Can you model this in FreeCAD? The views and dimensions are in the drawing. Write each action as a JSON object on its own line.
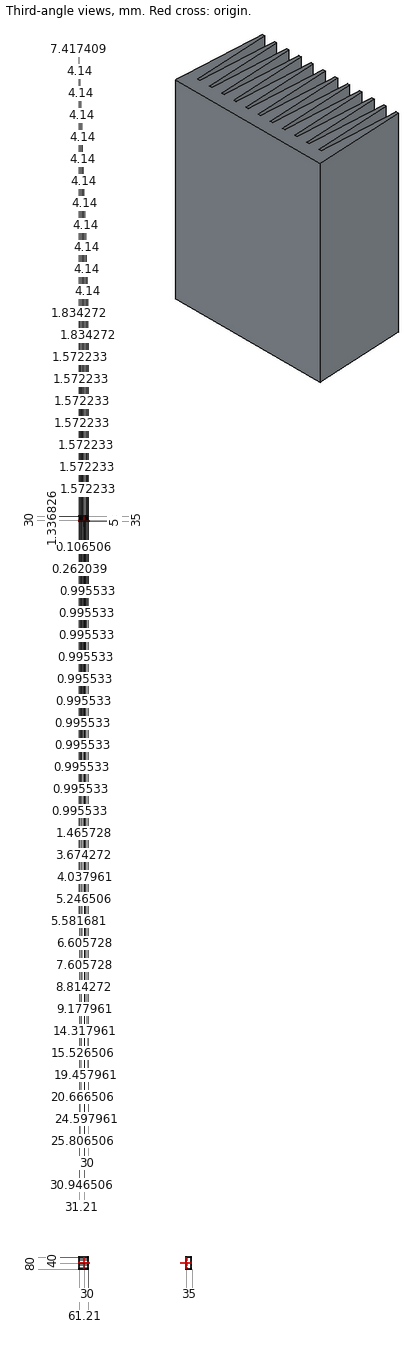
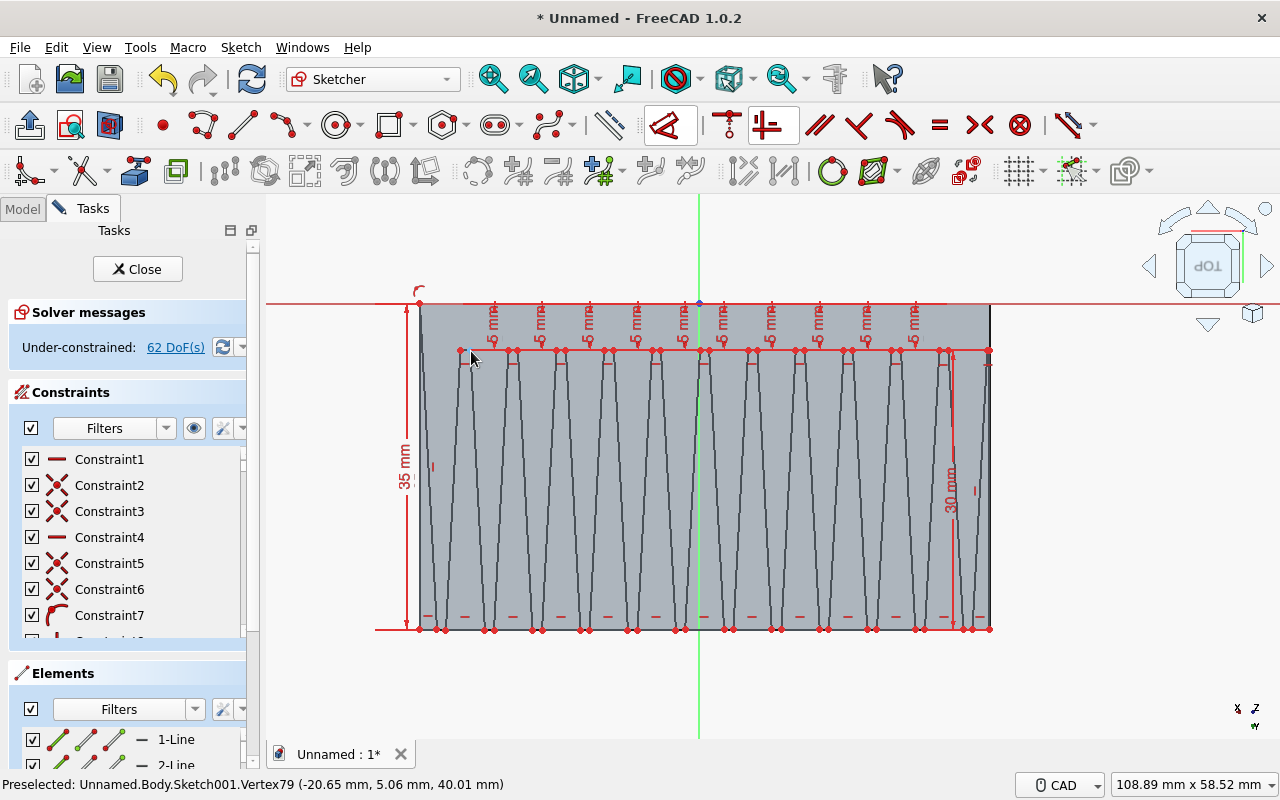
{"action": "scroll", "coordinate": [939, 351], "scroll_direction": "up", "scroll_amount": 2}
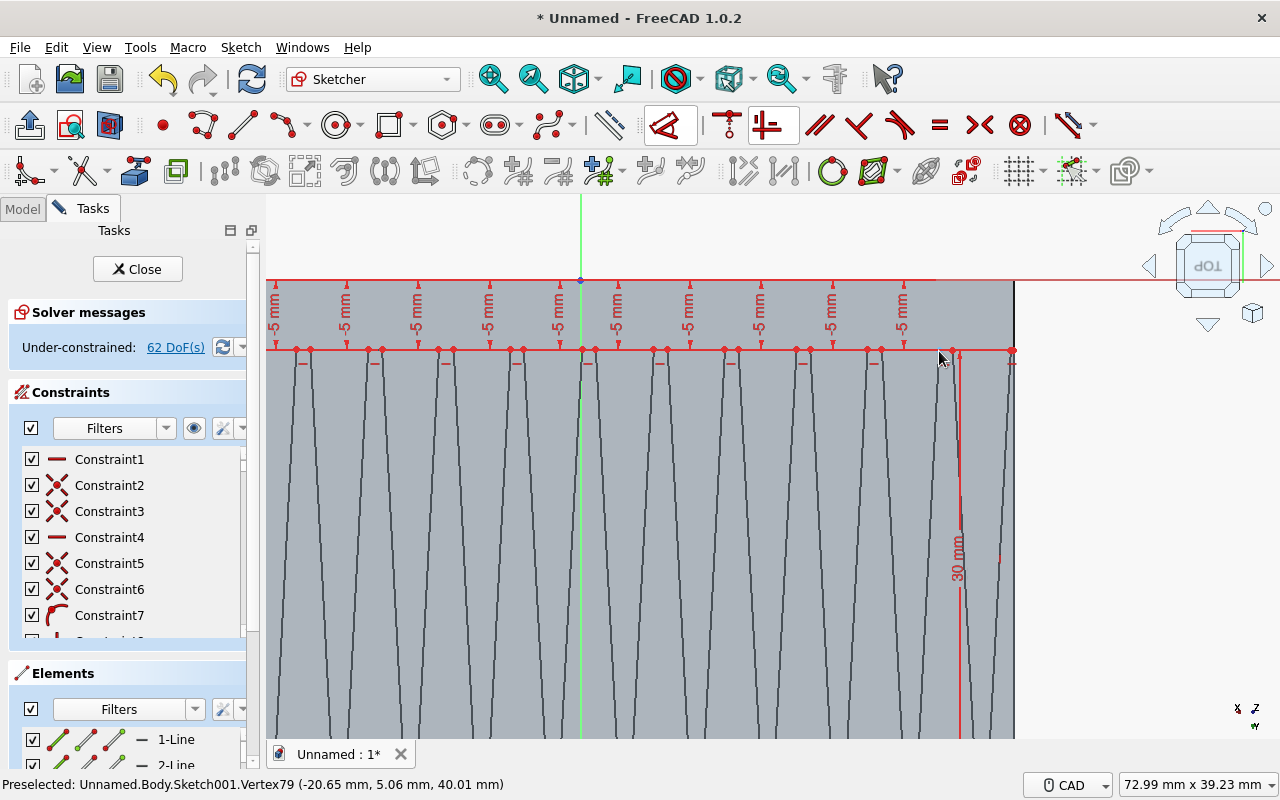
{"action": "left_click", "coordinate": [939, 350]}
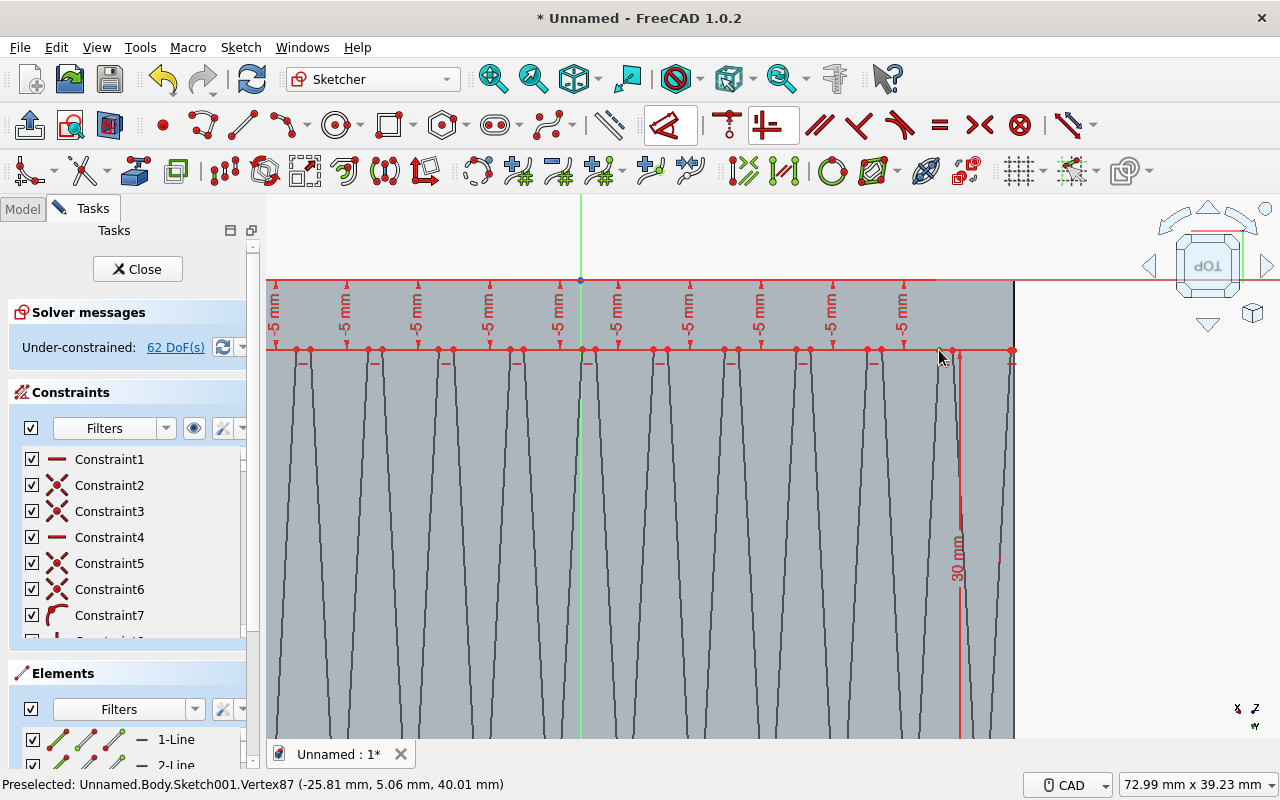
{"action": "key", "text": "i"}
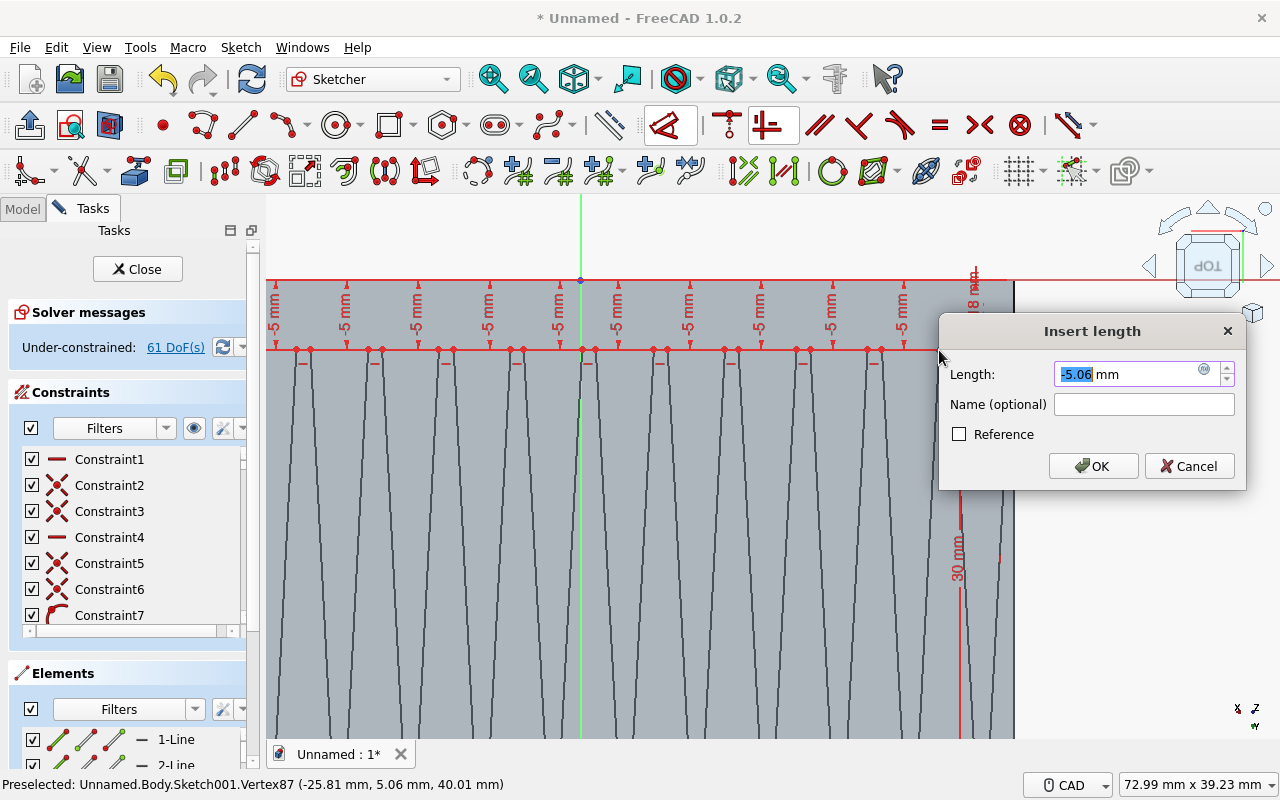
{"action": "type", "text": "-5"}
{"action": "key", "text": "Return"}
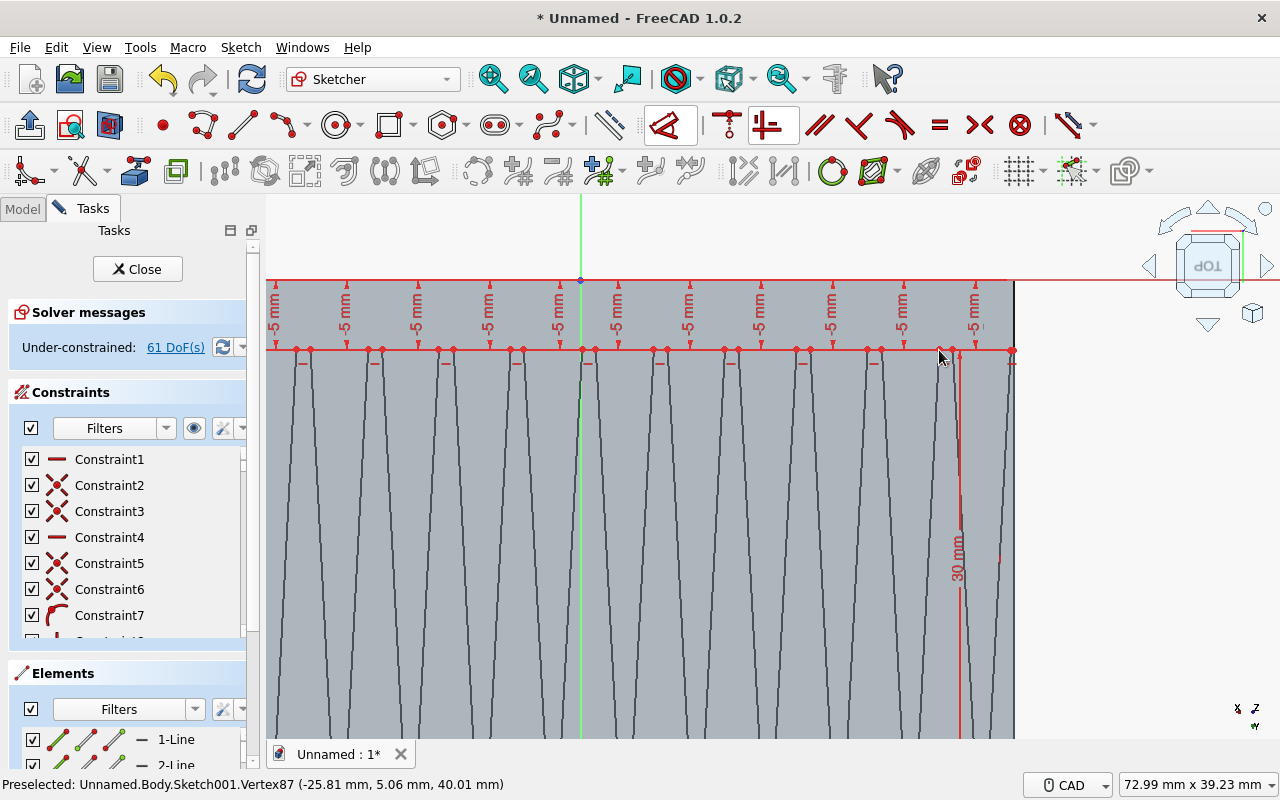
{"action": "scroll", "coordinate": [1011, 350], "scroll_direction": "up", "scroll_amount": 7}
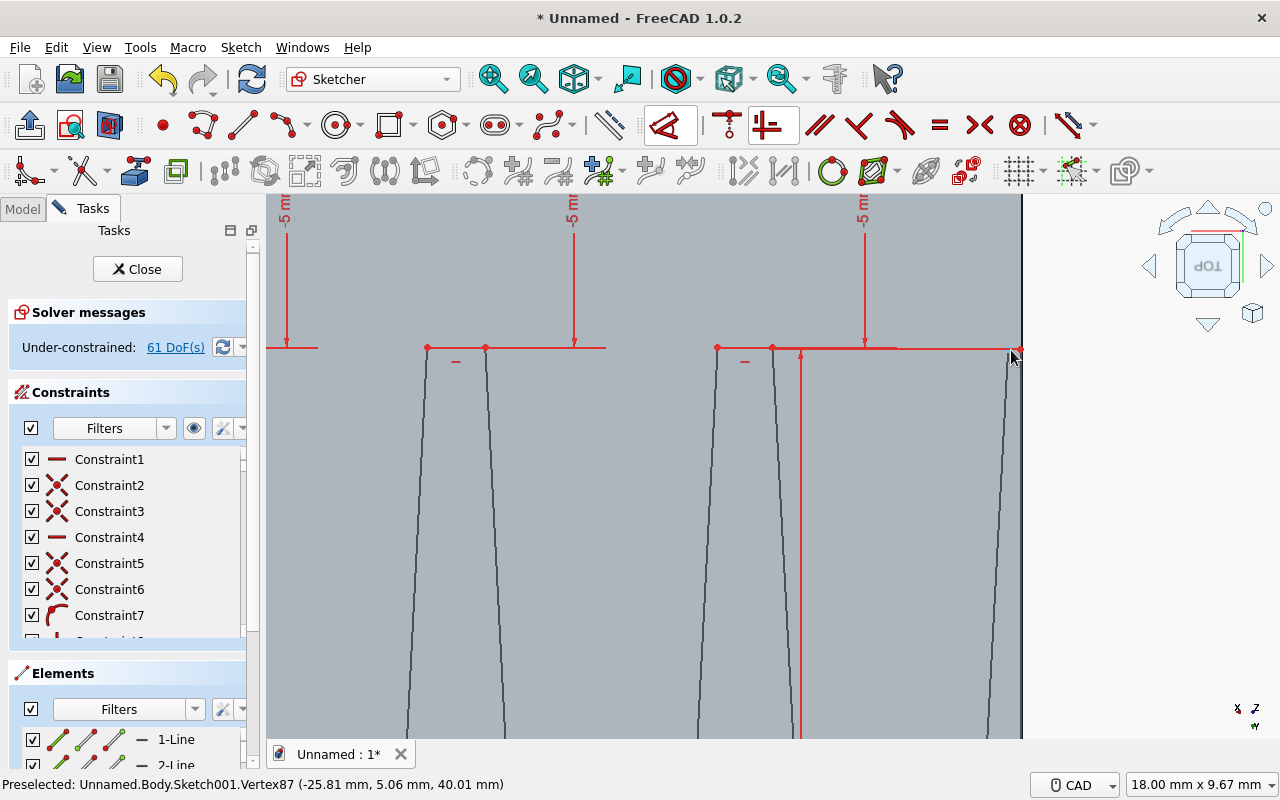
{"action": "left_click", "coordinate": [1008, 349]}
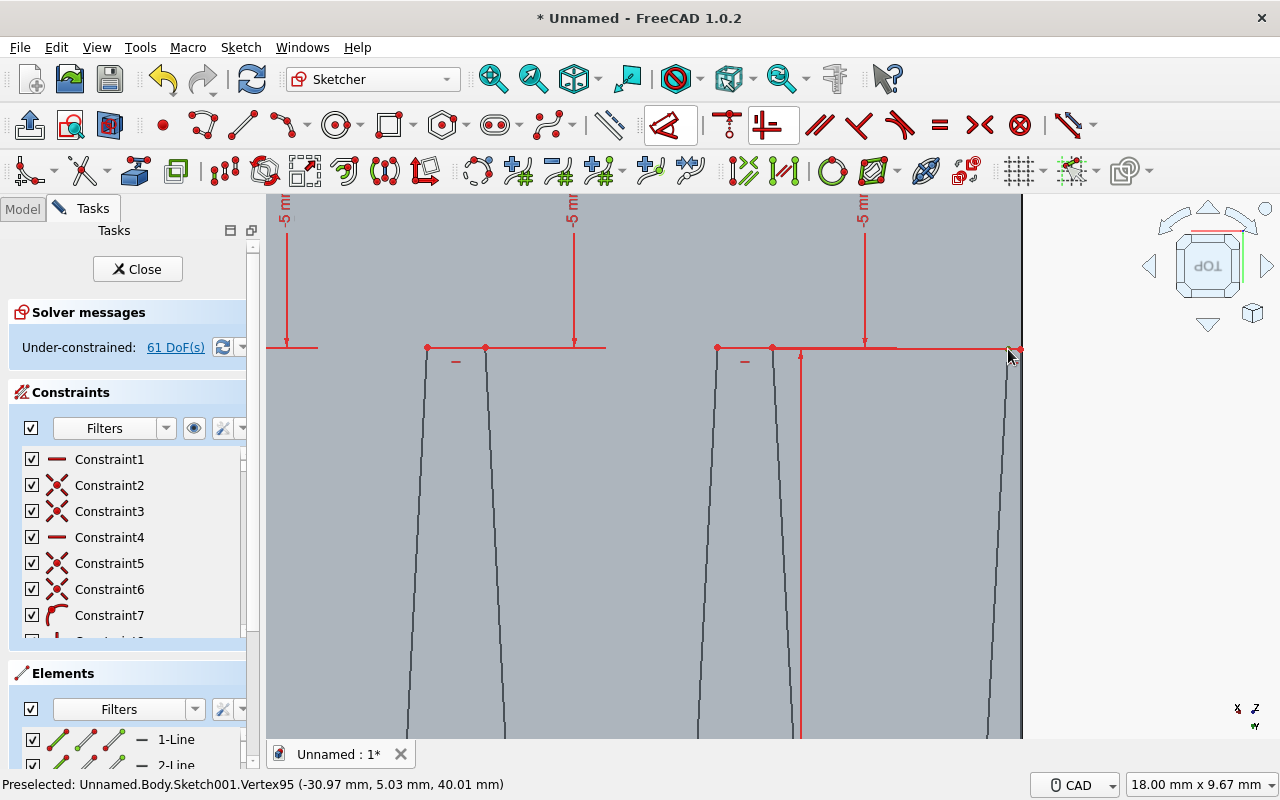
{"action": "key", "text": "i"}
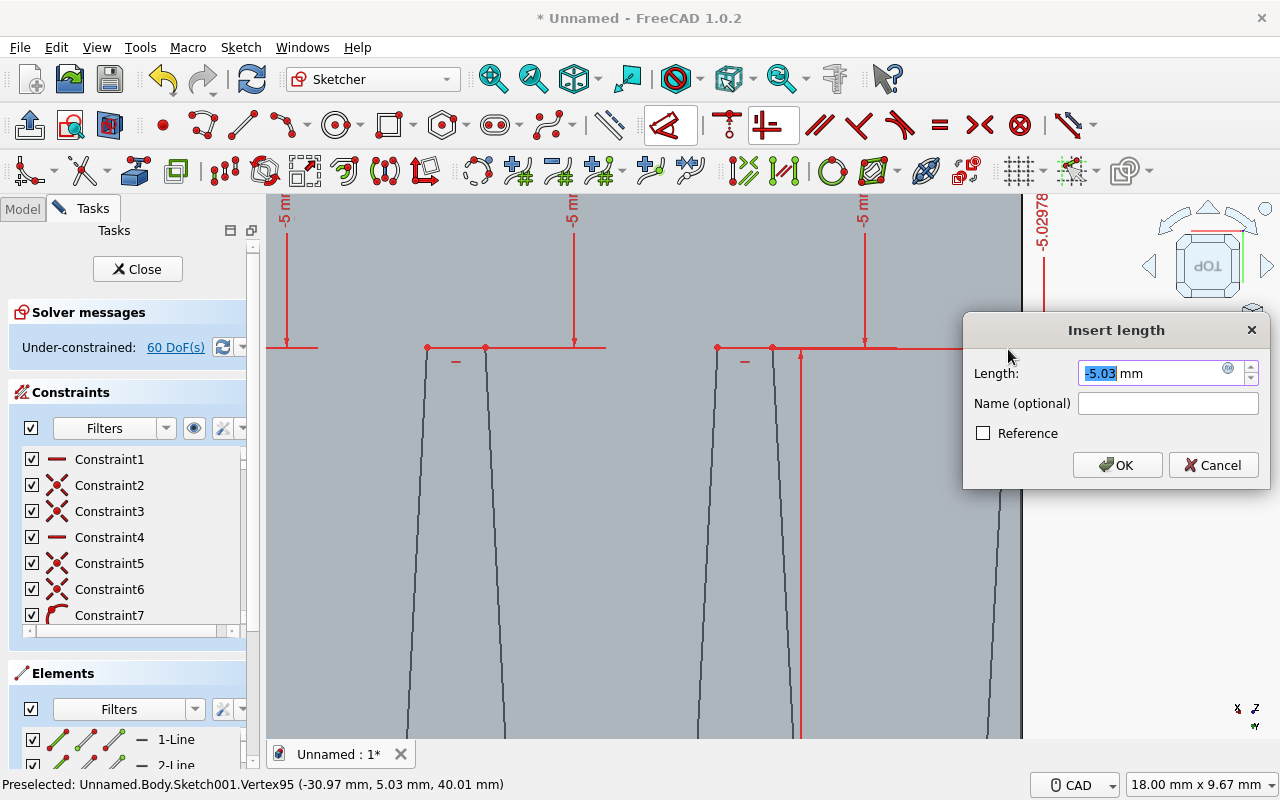
{"action": "type", "text": "-5"}
{"action": "key", "text": "Return"}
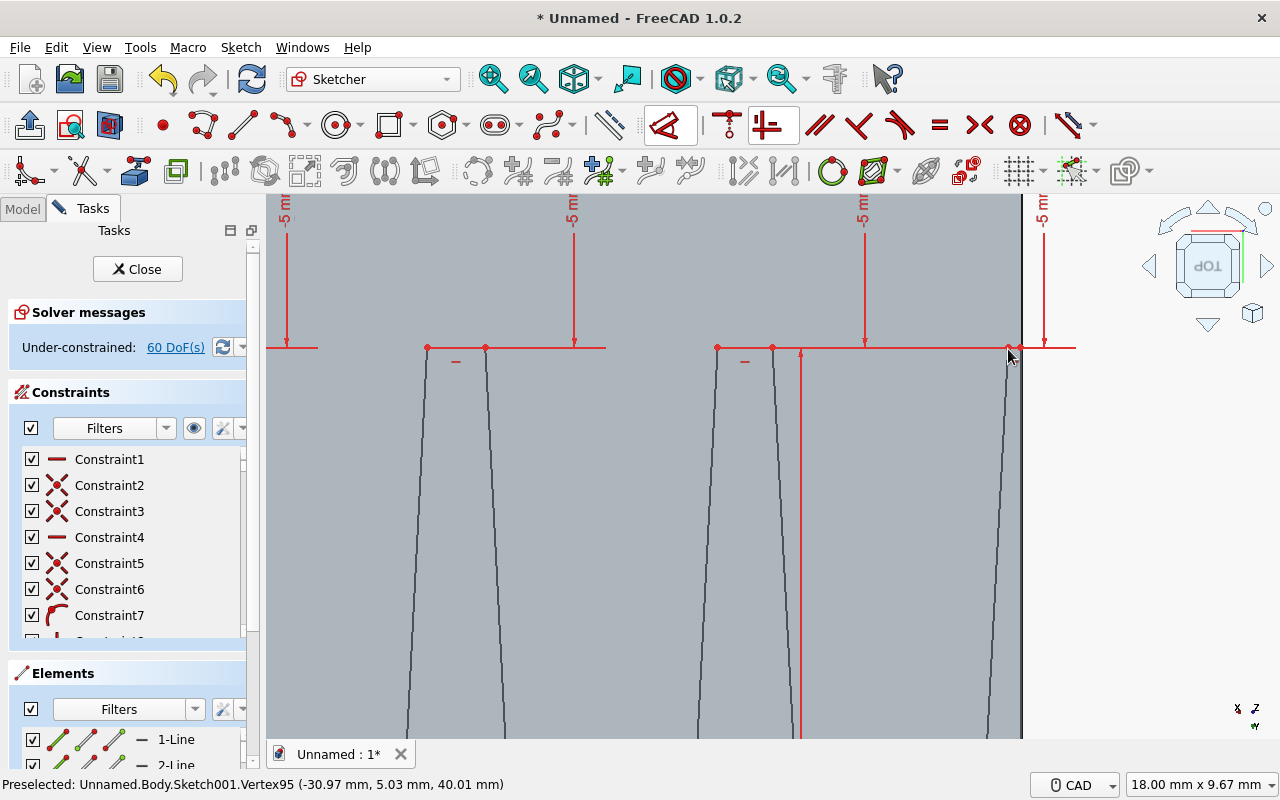
{"action": "scroll", "coordinate": [983, 351], "scroll_direction": "down", "scroll_amount": 9}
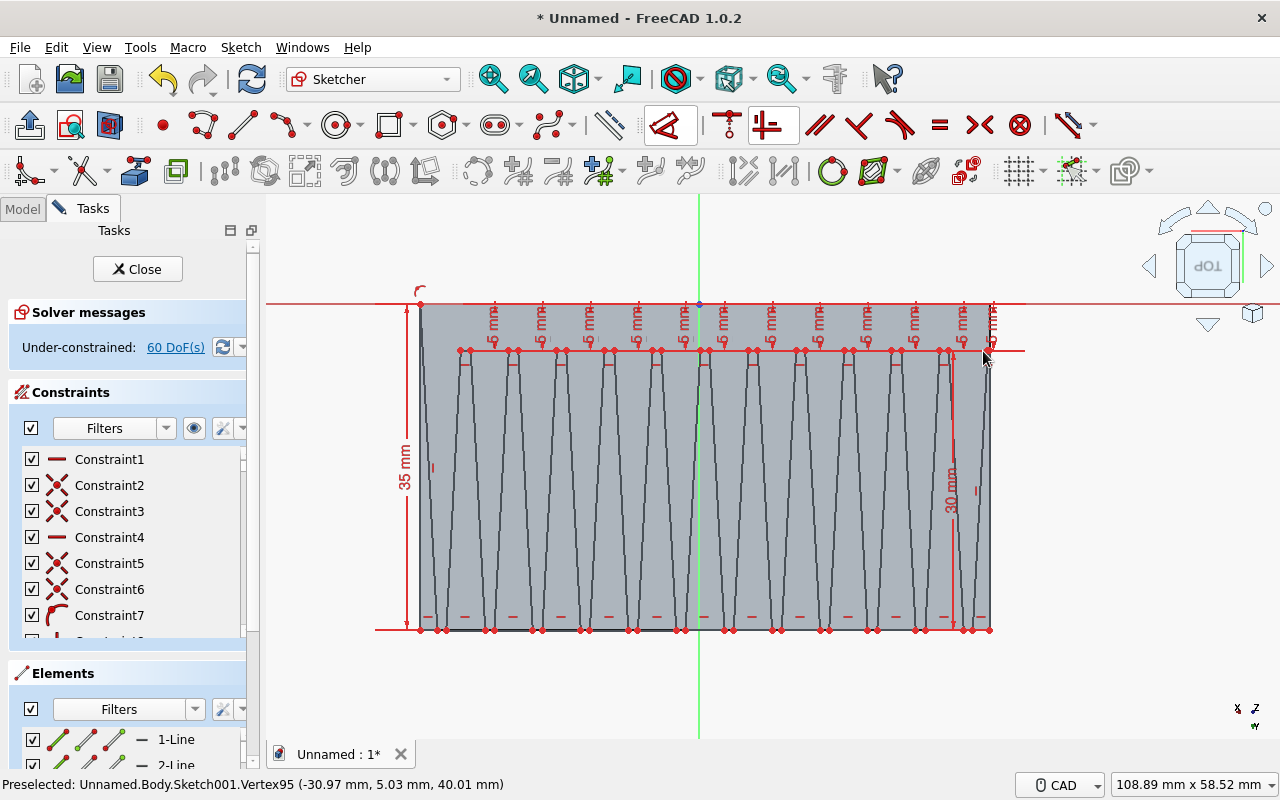
{"action": "scroll", "coordinate": [446, 631], "scroll_direction": "up", "scroll_amount": 2}